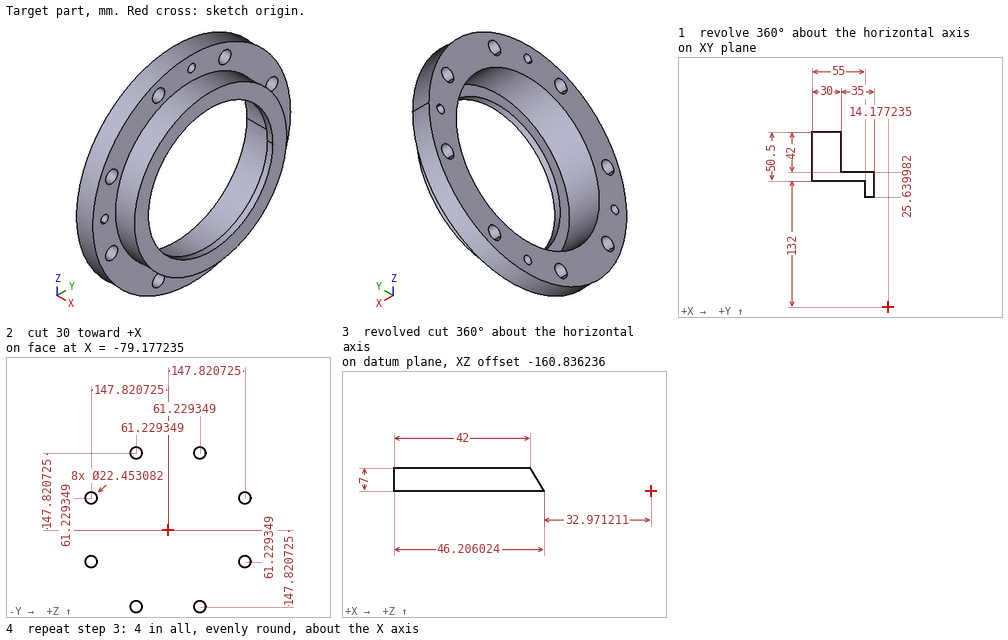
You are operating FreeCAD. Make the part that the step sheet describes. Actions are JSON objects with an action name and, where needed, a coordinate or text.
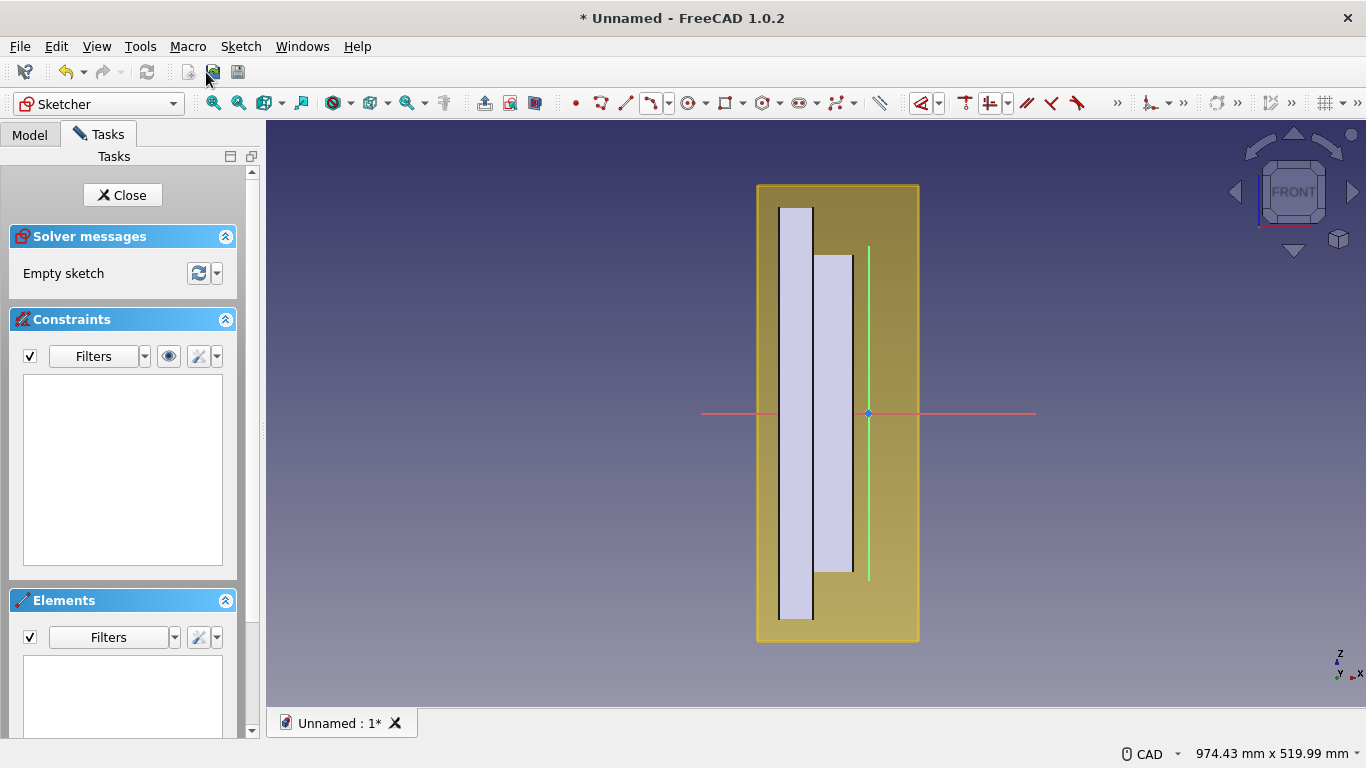
{"action": "left_click", "coordinate": [535, 104]}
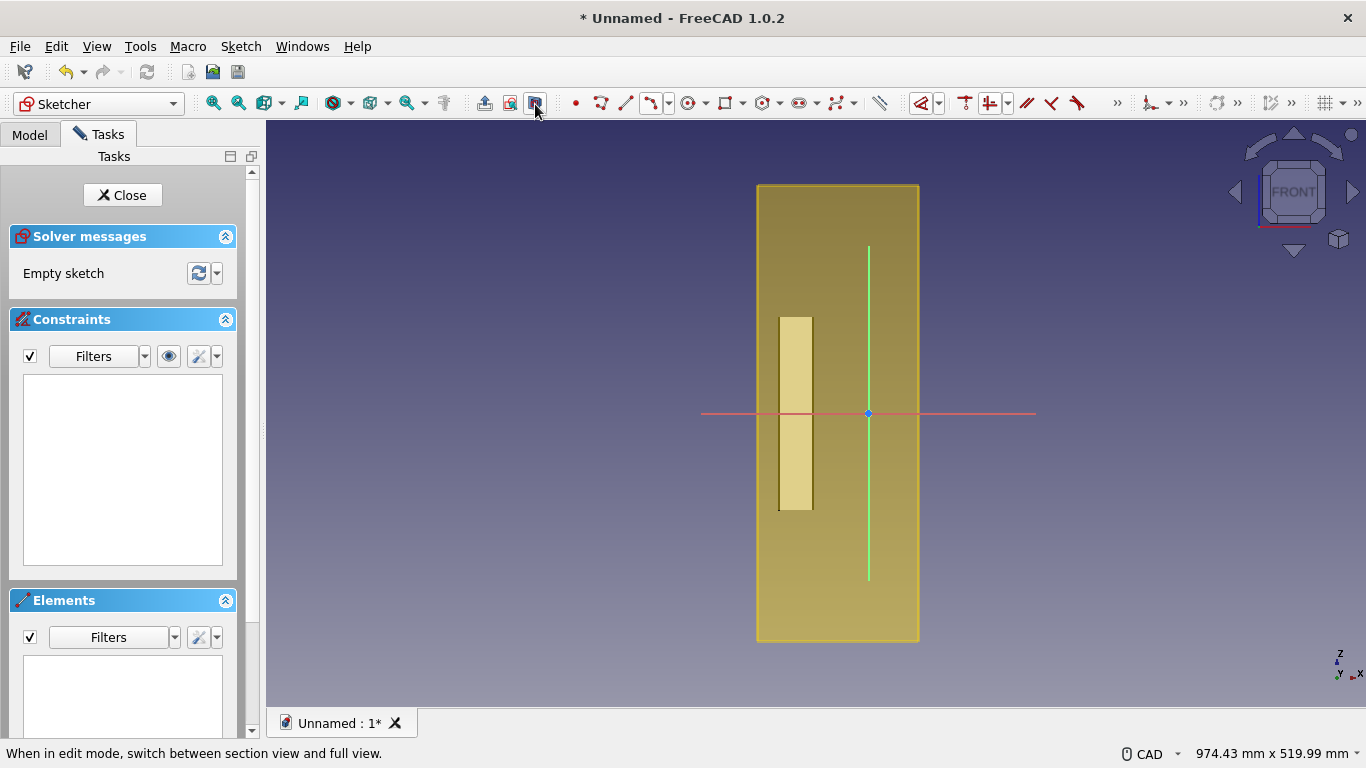
{"action": "scroll", "coordinate": [836, 409], "scroll_direction": "up", "scroll_amount": 10}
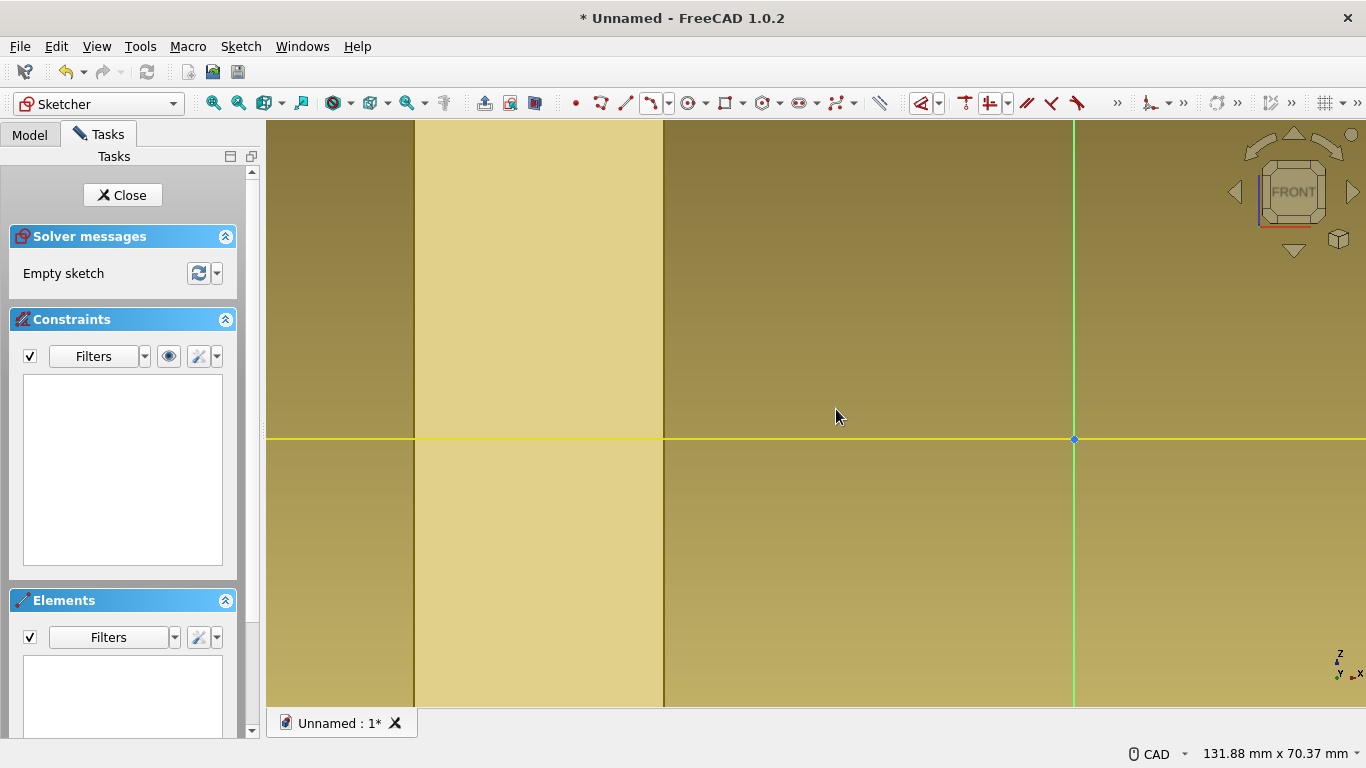
{"action": "left_click", "coordinate": [601, 104]}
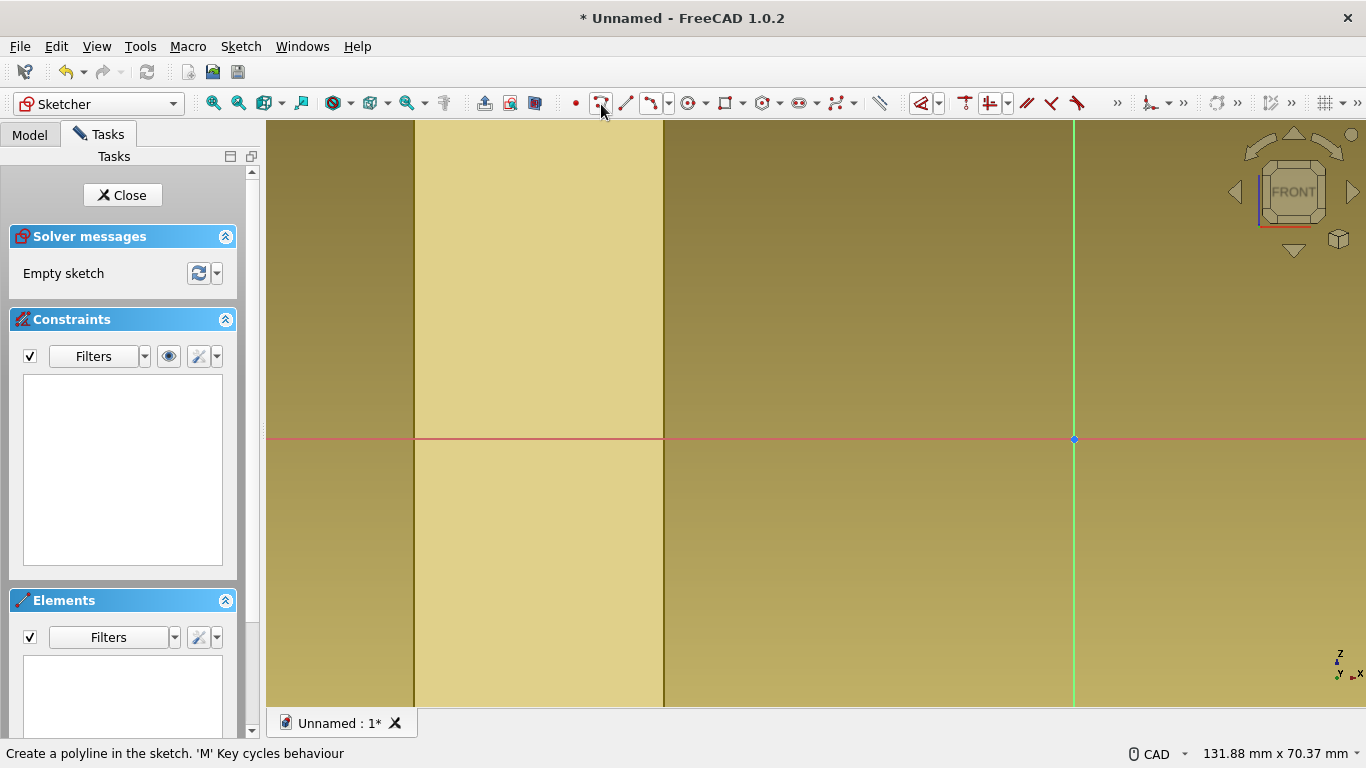
{"action": "left_click", "coordinate": [799, 439]}
{"action": "left_click", "coordinate": [414, 430]}
{"action": "left_click", "coordinate": [414, 381]}
{"action": "left_click", "coordinate": [764, 381]}
{"action": "left_click", "coordinate": [799, 439]}
{"action": "key", "text": "Escape"}
{"action": "key", "text": "Escape"}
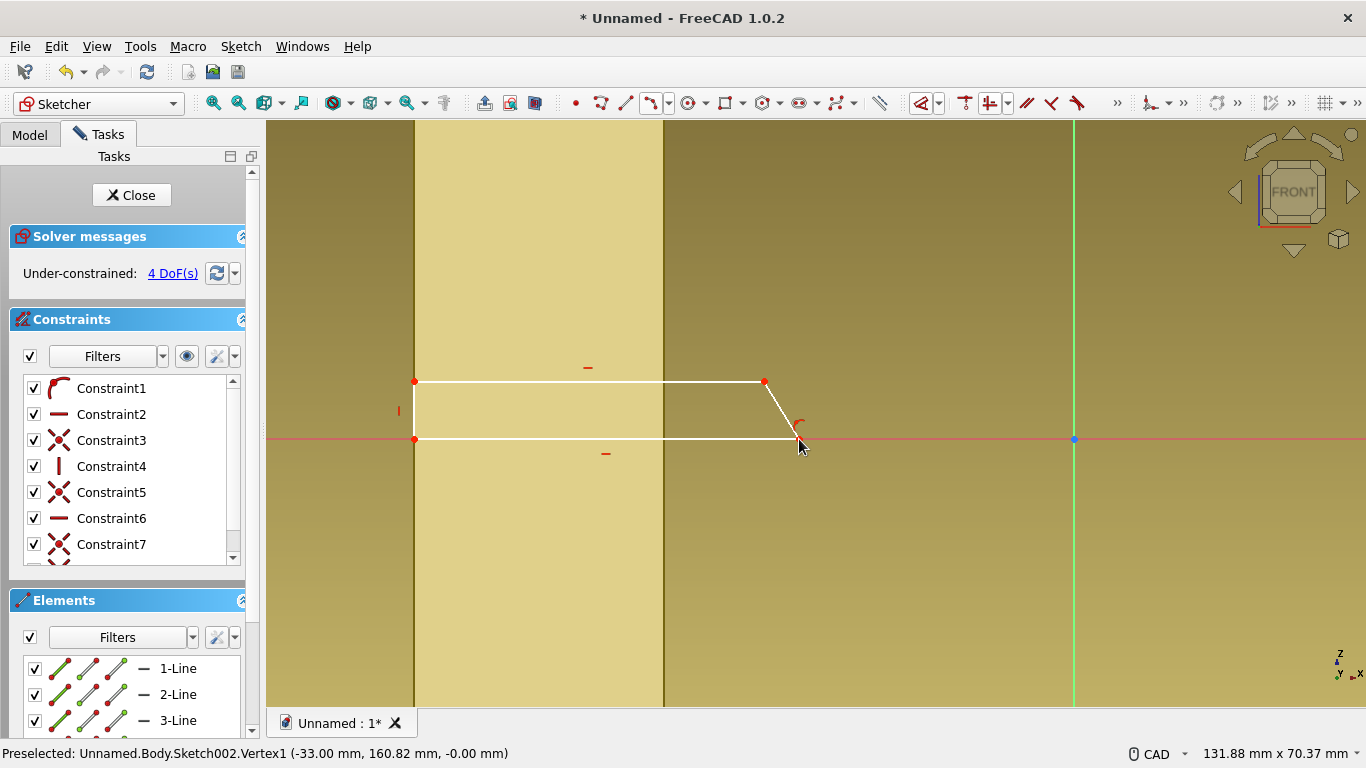
{"action": "left_click", "coordinate": [414, 422]}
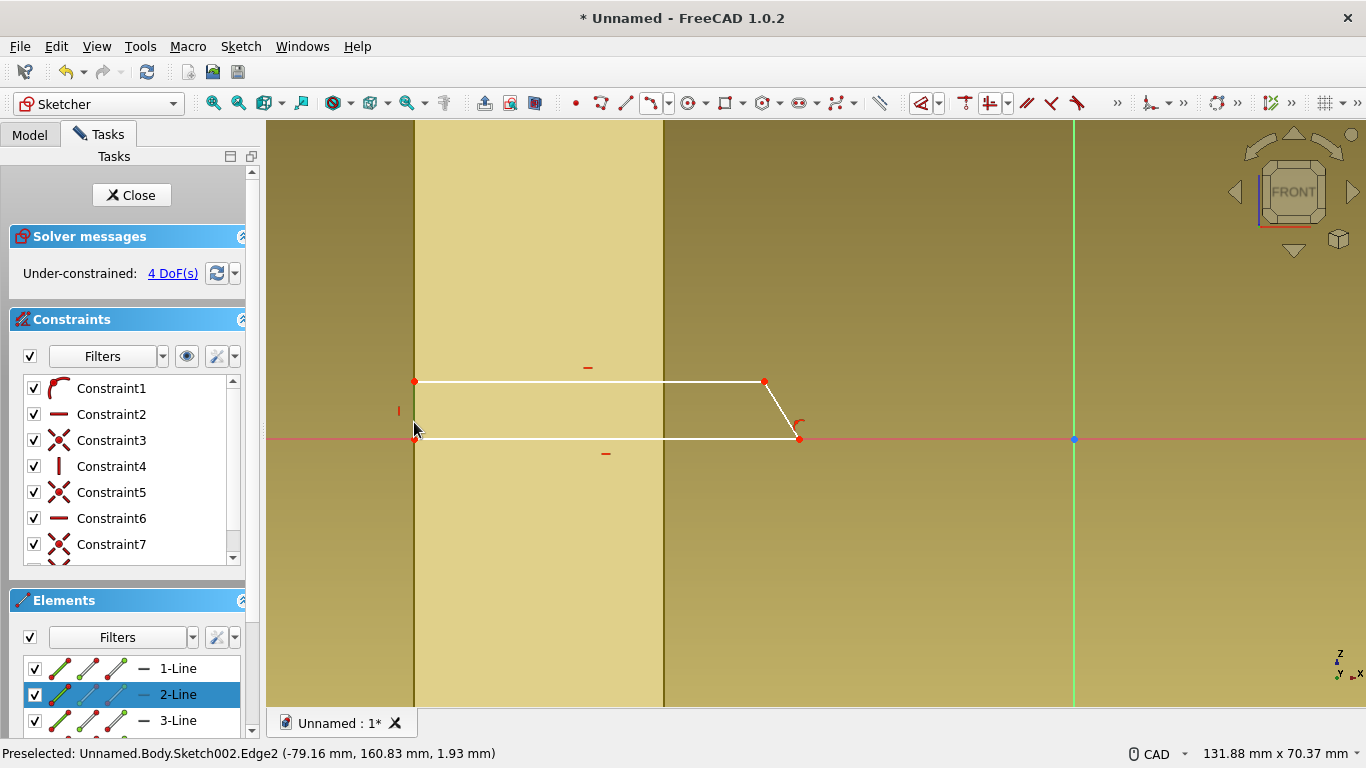
{"action": "key", "text": "i"}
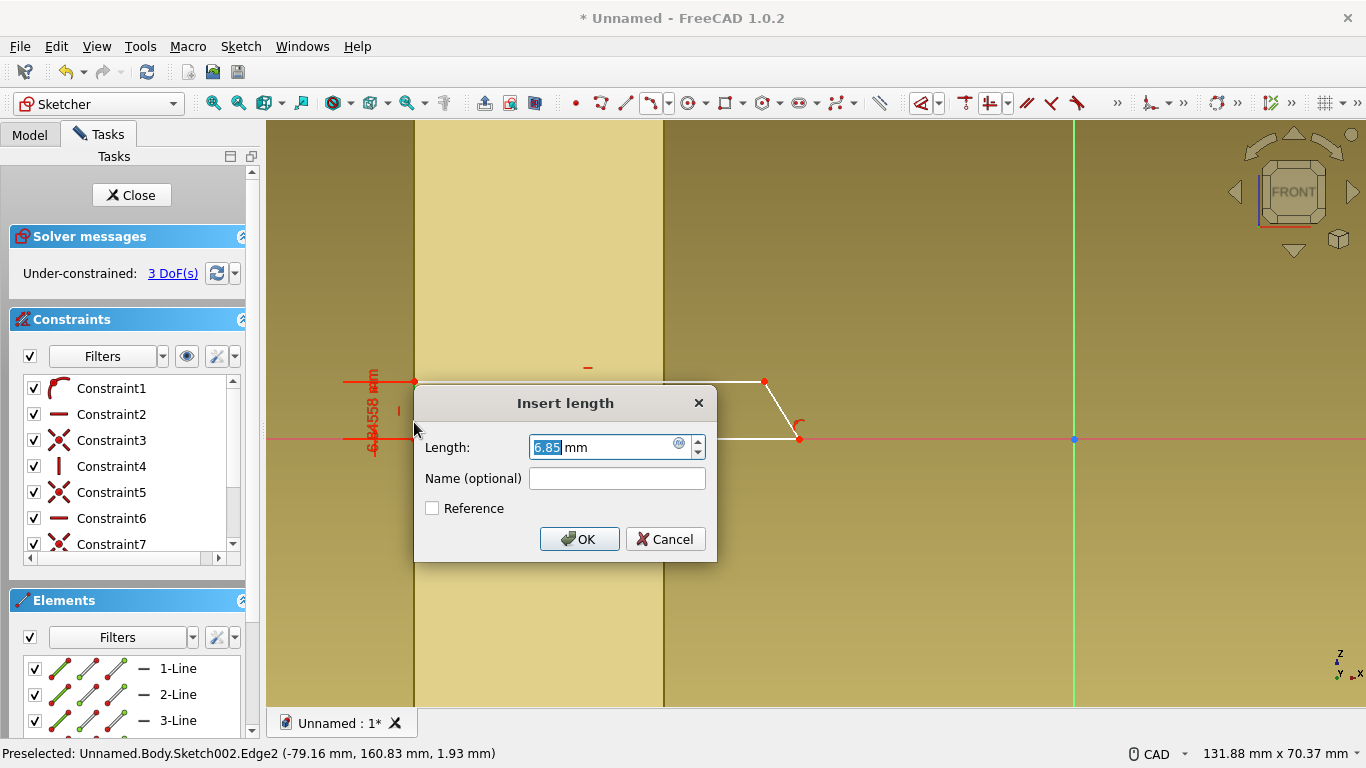
{"action": "type", "text": "7"}
{"action": "key", "text": "Return"}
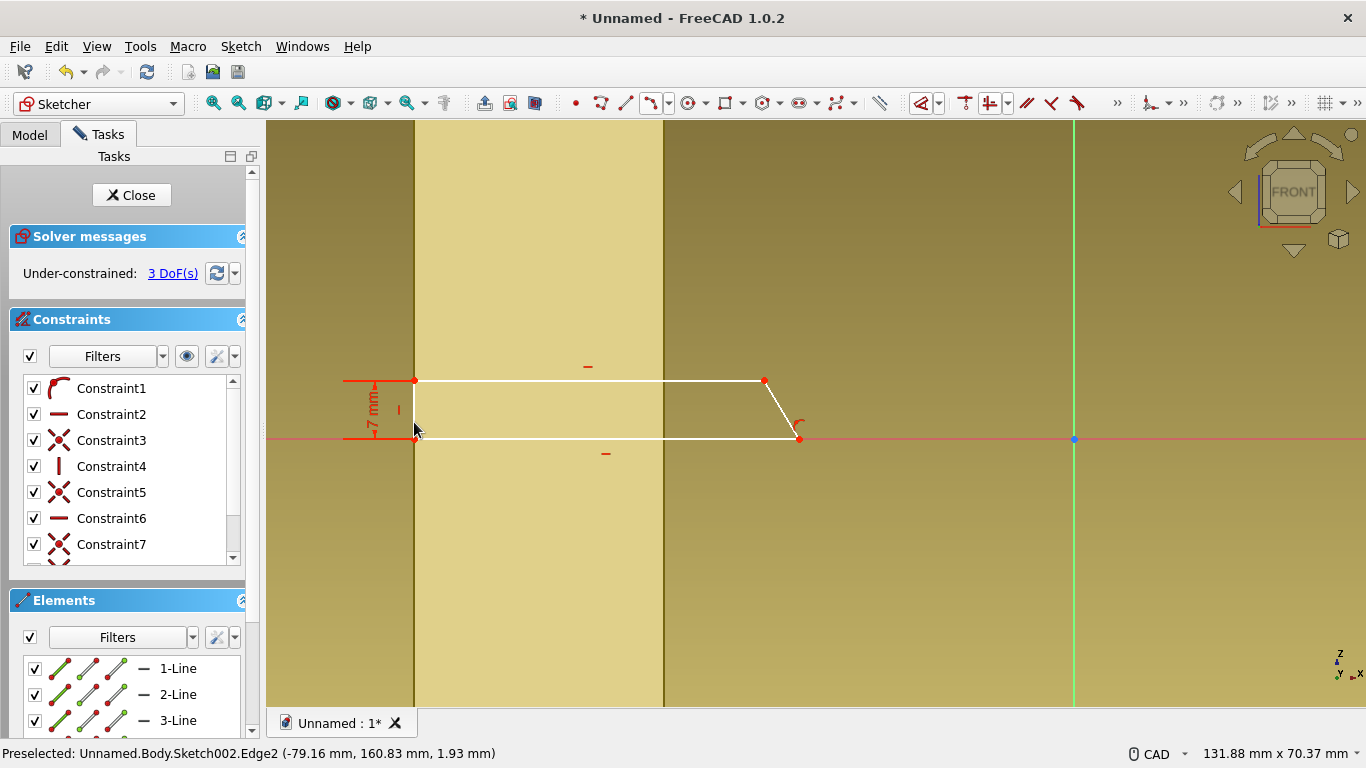
{"action": "left_click", "coordinate": [519, 381]}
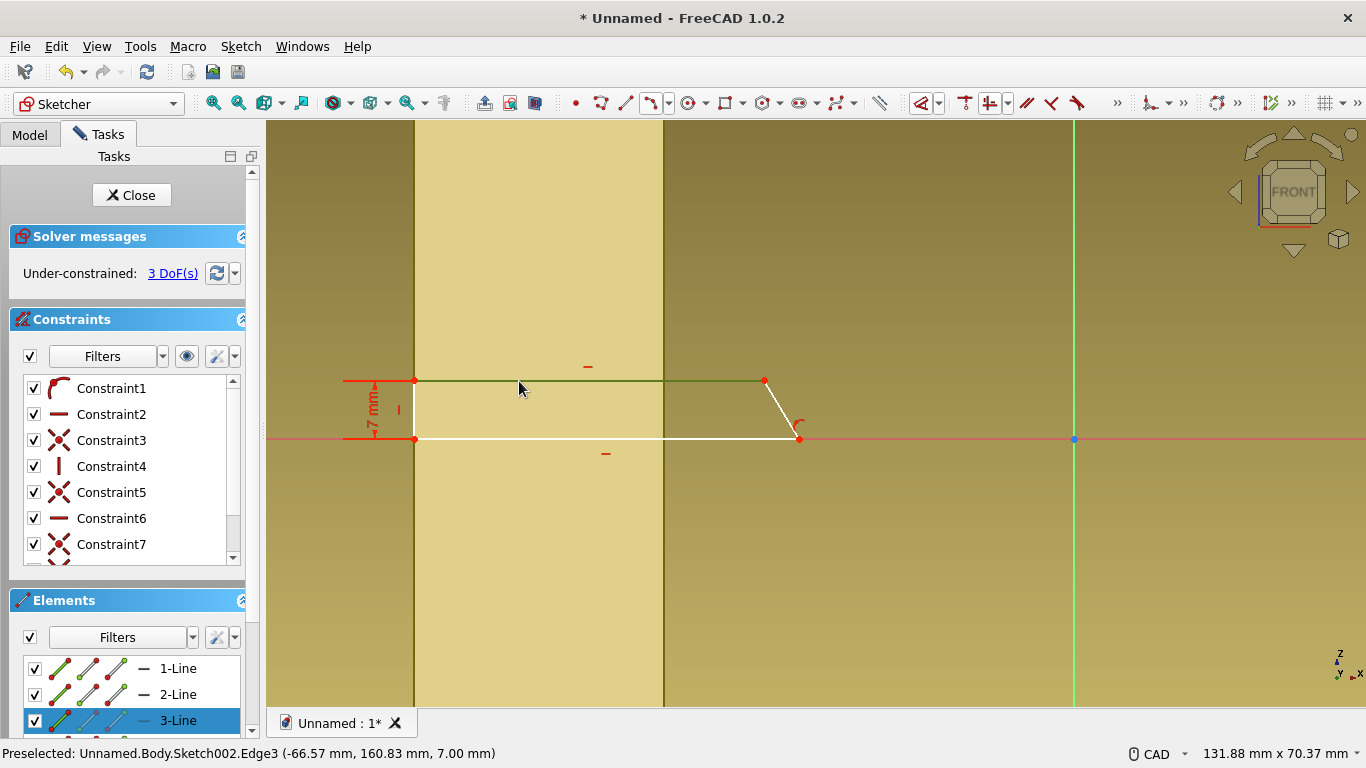
{"action": "left_click", "coordinate": [938, 104]}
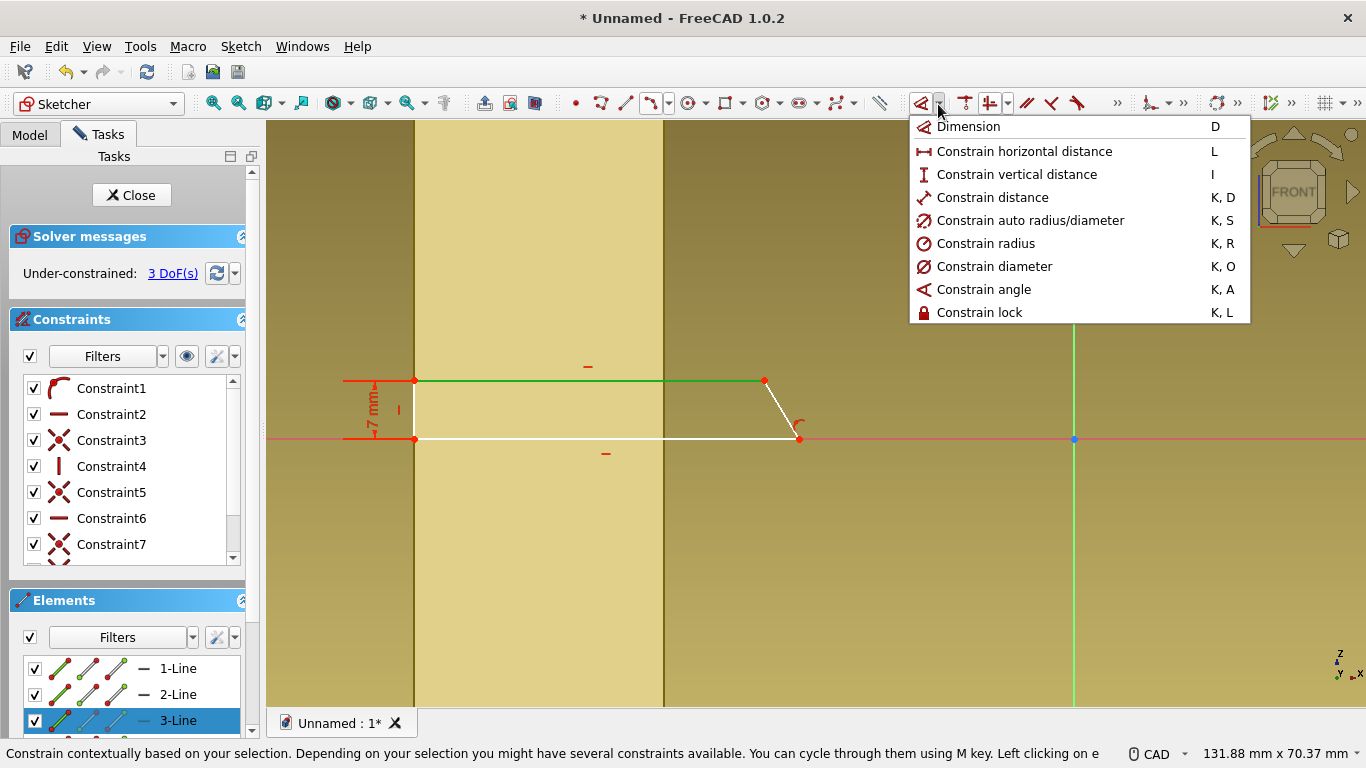
{"action": "left_click", "coordinate": [1080, 152]}